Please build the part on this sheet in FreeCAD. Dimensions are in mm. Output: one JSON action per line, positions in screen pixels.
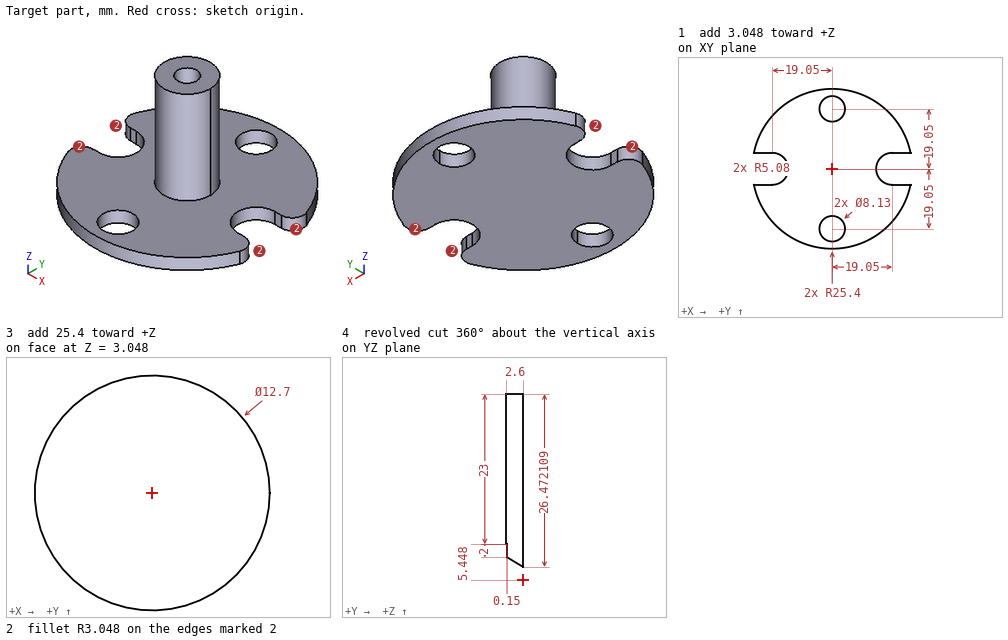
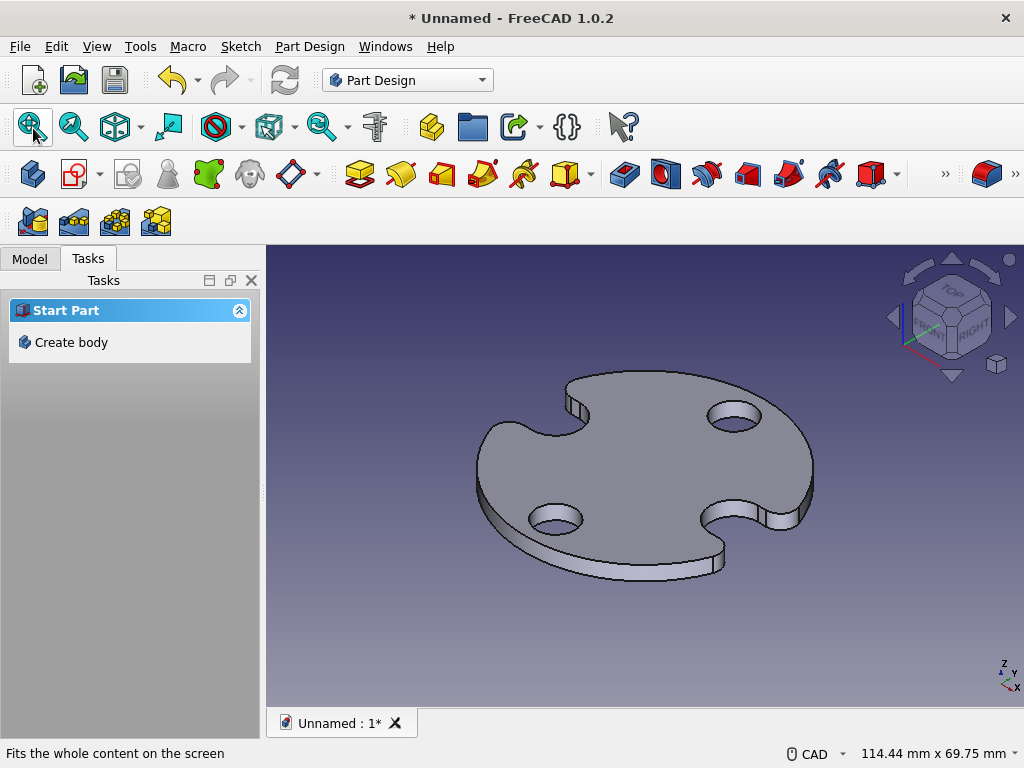
{"action": "left_click", "coordinate": [645, 467]}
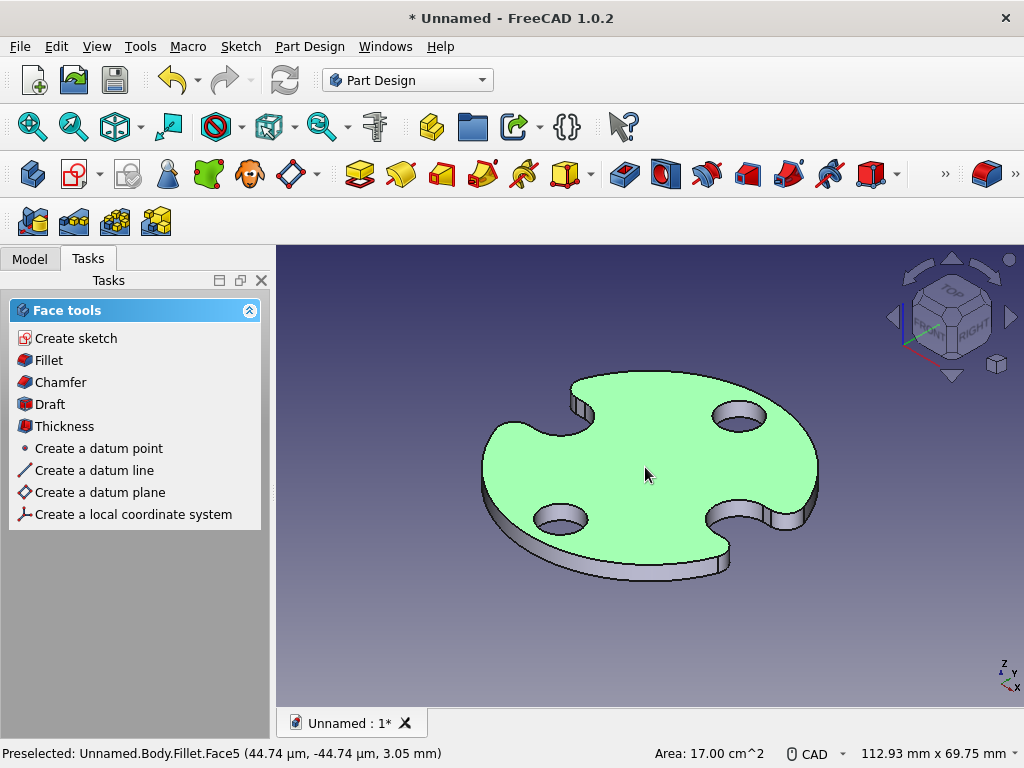
{"action": "left_click", "coordinate": [74, 174]}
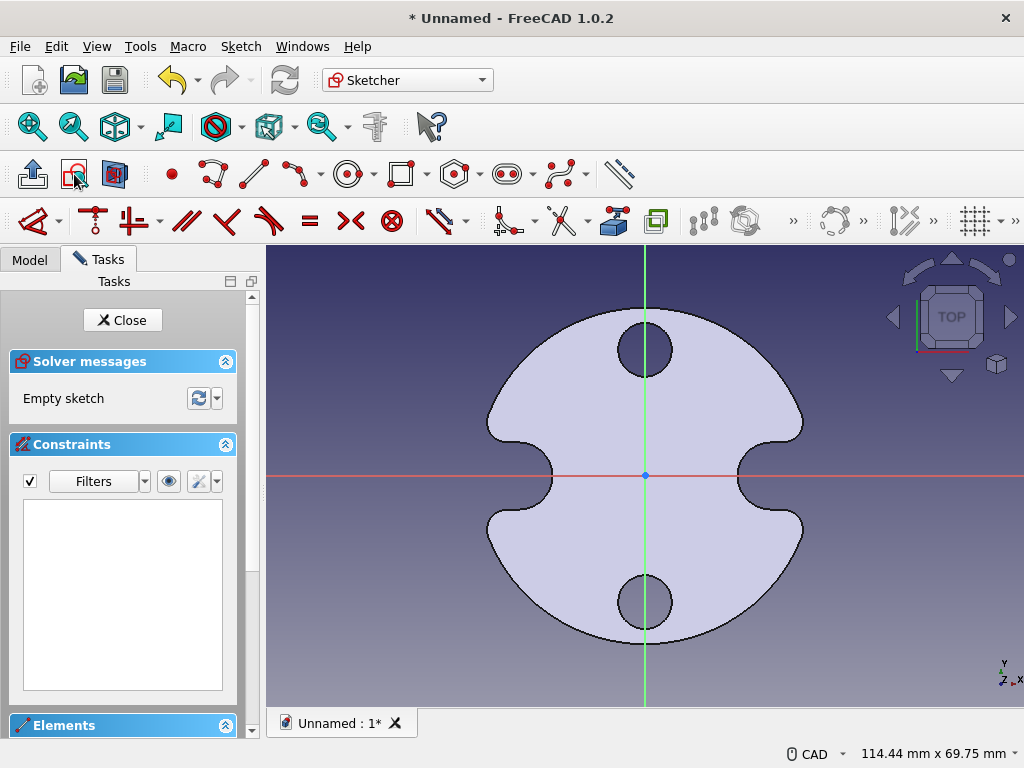
{"action": "scroll", "coordinate": [675, 476], "scroll_direction": "up", "scroll_amount": 6}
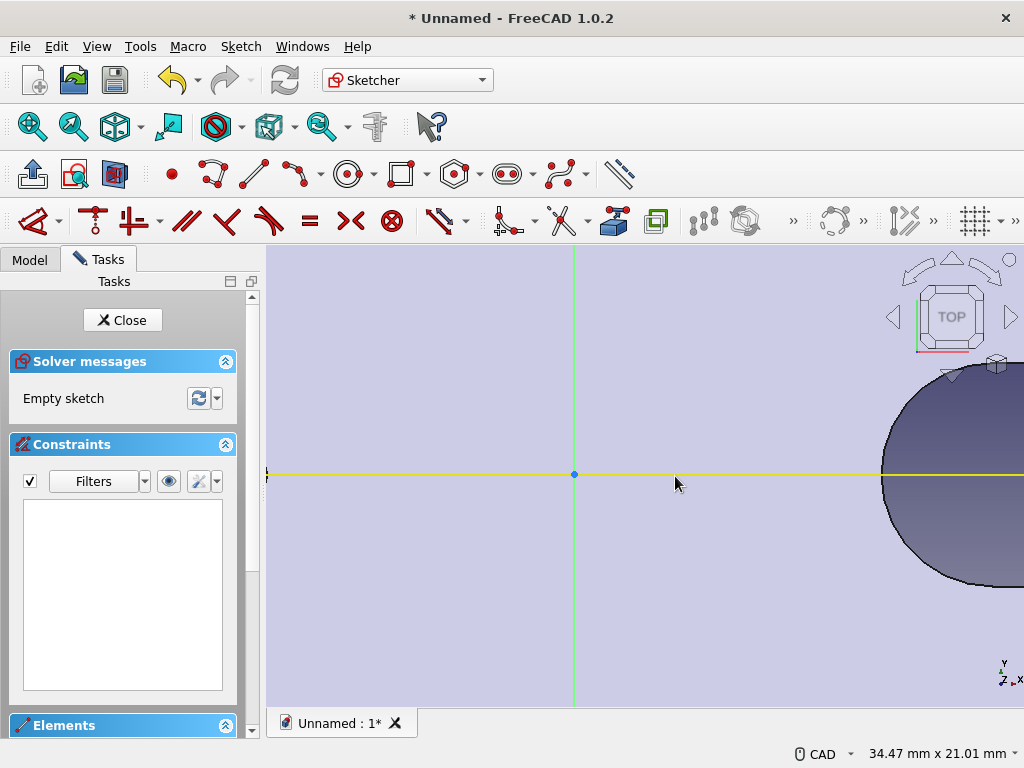
{"action": "left_click", "coordinate": [348, 174]}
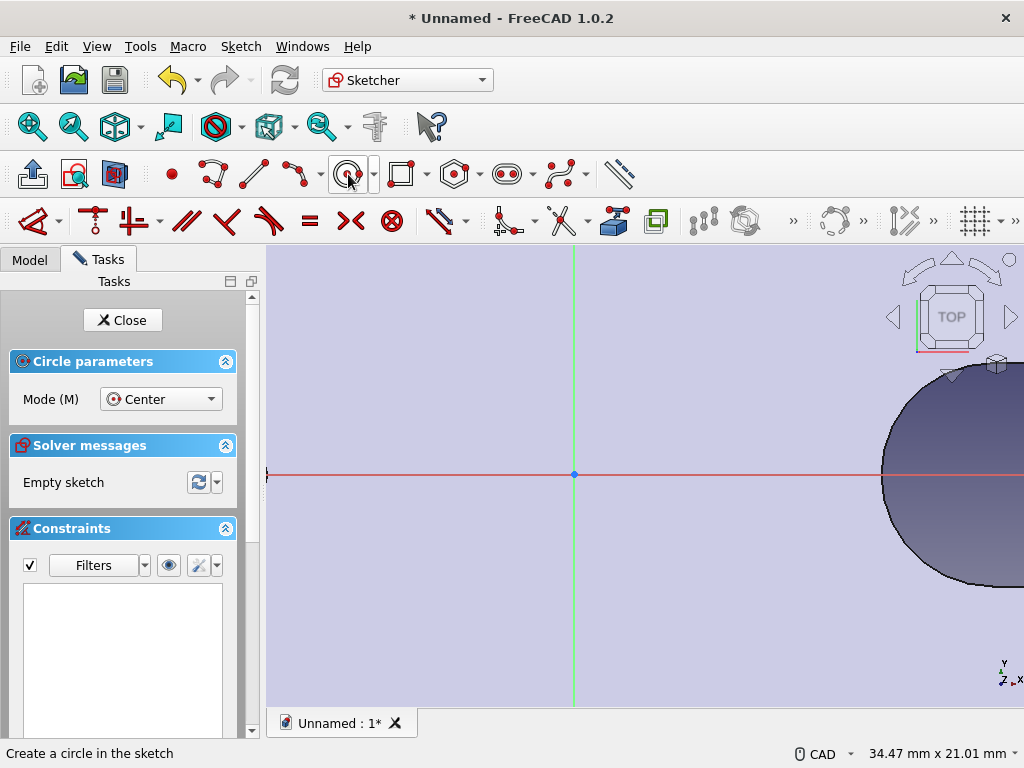
{"action": "left_click", "coordinate": [574, 475]}
{"action": "mouse_move", "coordinate": [673, 376]}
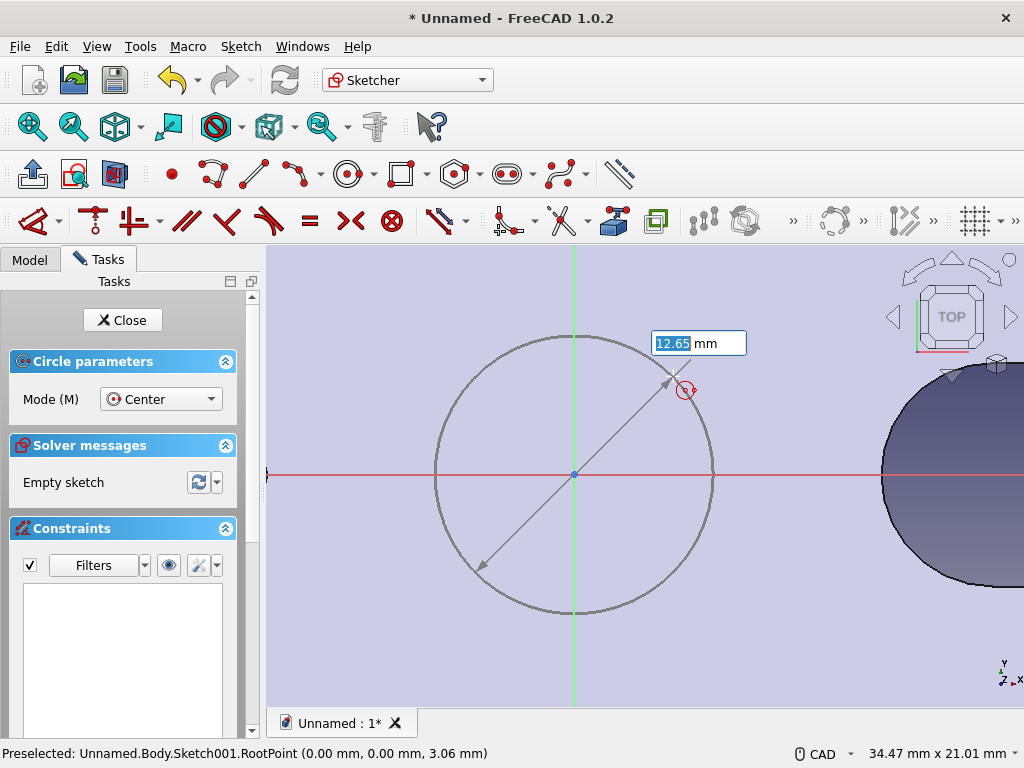
{"action": "type", "text": "12.7"}
{"action": "key", "text": "Return"}
{"action": "key", "text": "Escape"}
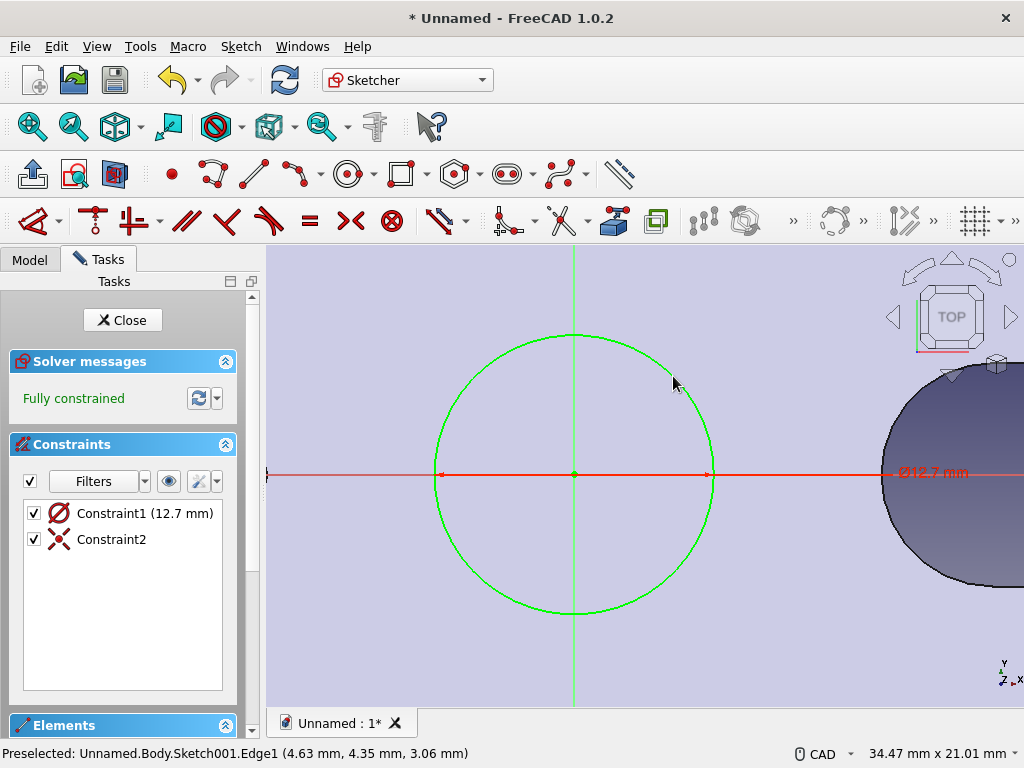
{"action": "left_click", "coordinate": [123, 320]}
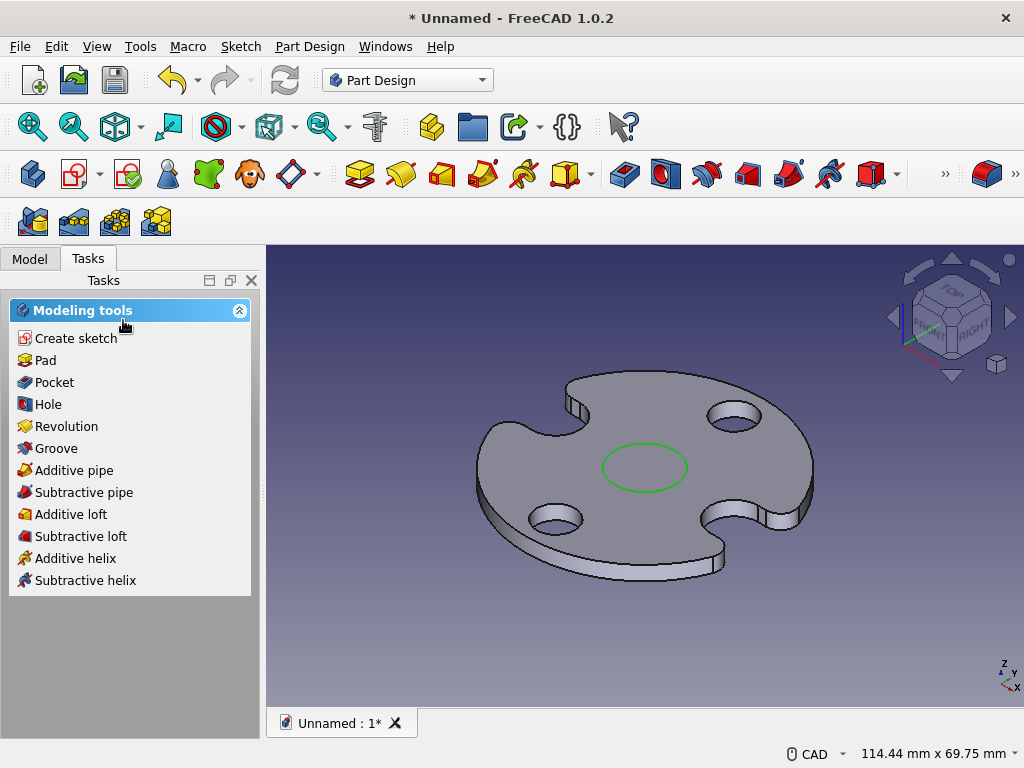
{"action": "left_click", "coordinate": [360, 174]}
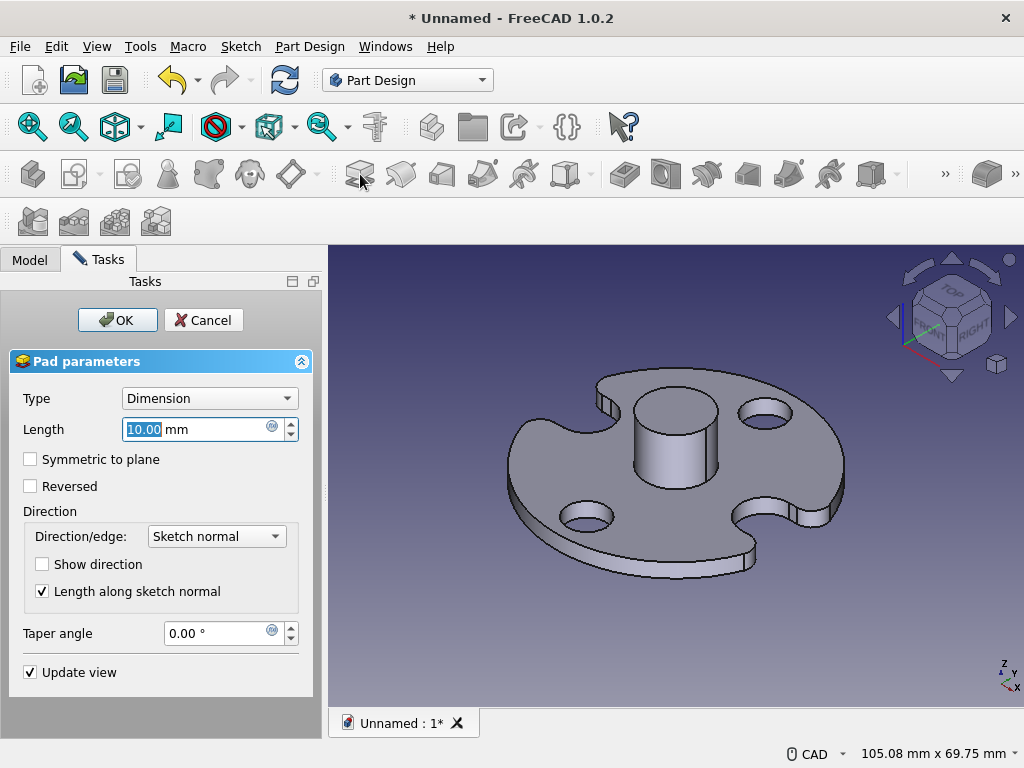
{"action": "type", "text": "25.4"}
{"action": "key", "text": "Tab"}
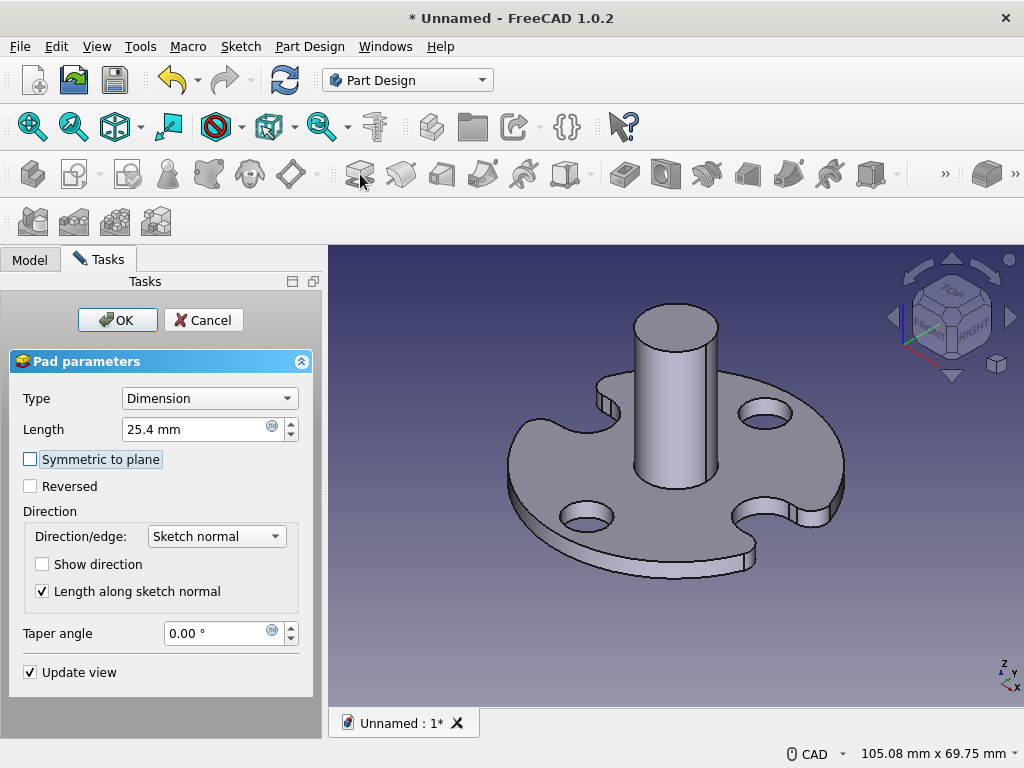
{"action": "left_click", "coordinate": [118, 320]}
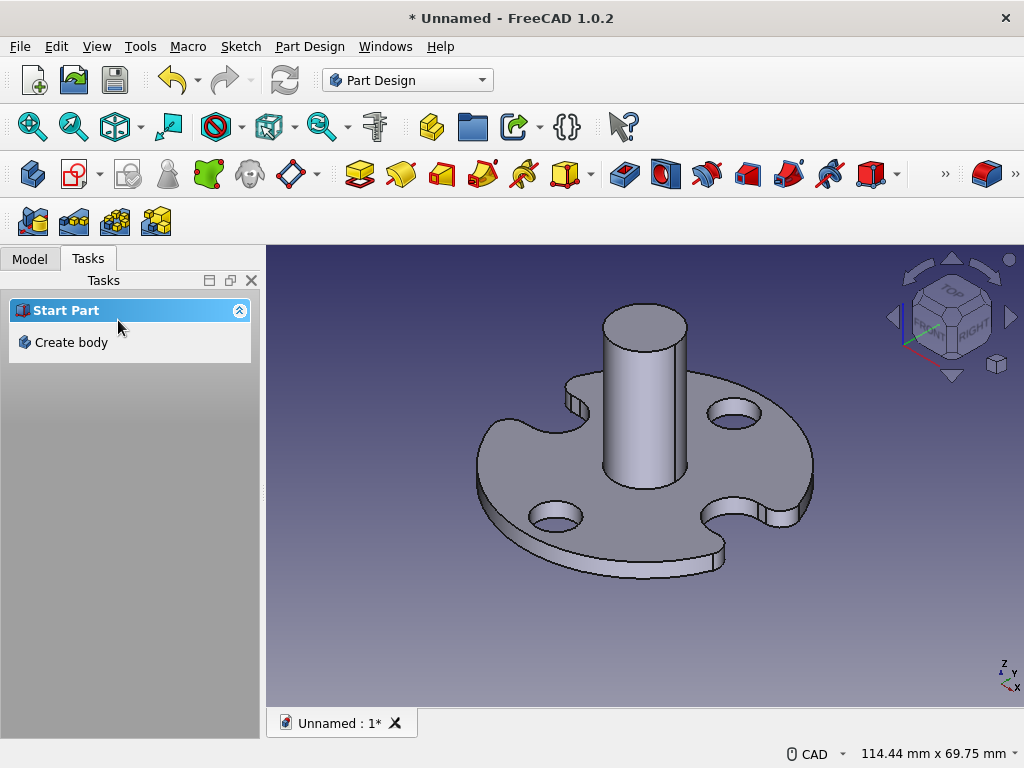
{"action": "left_click", "coordinate": [33, 128]}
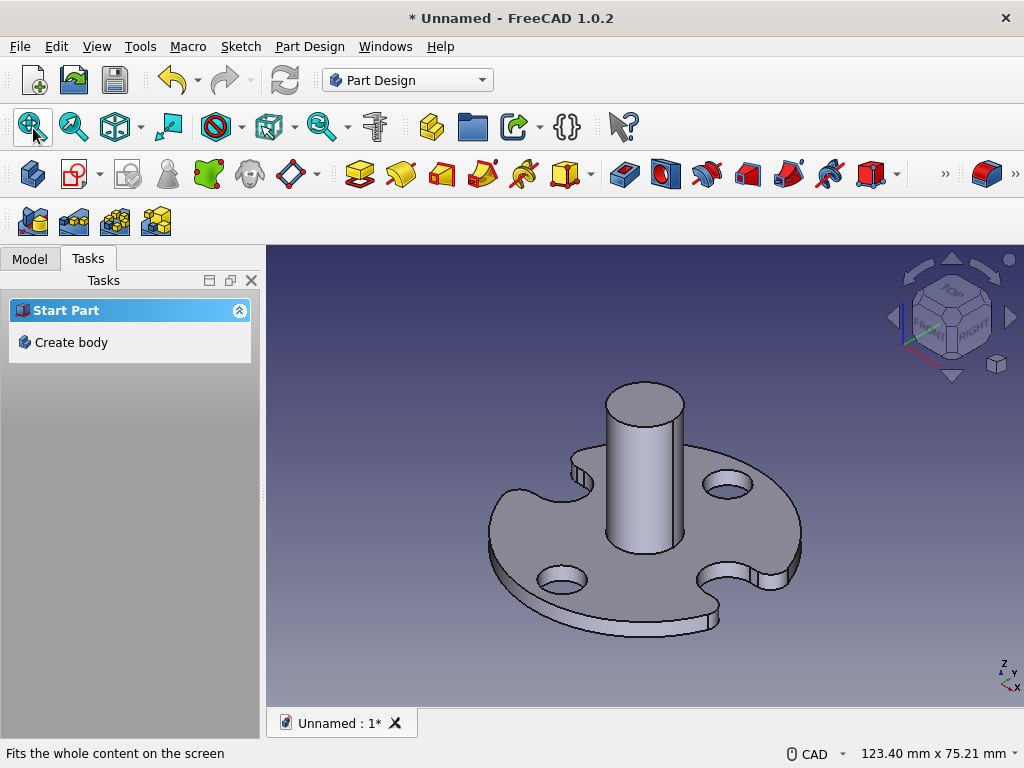
{"action": "left_click", "coordinate": [74, 174]}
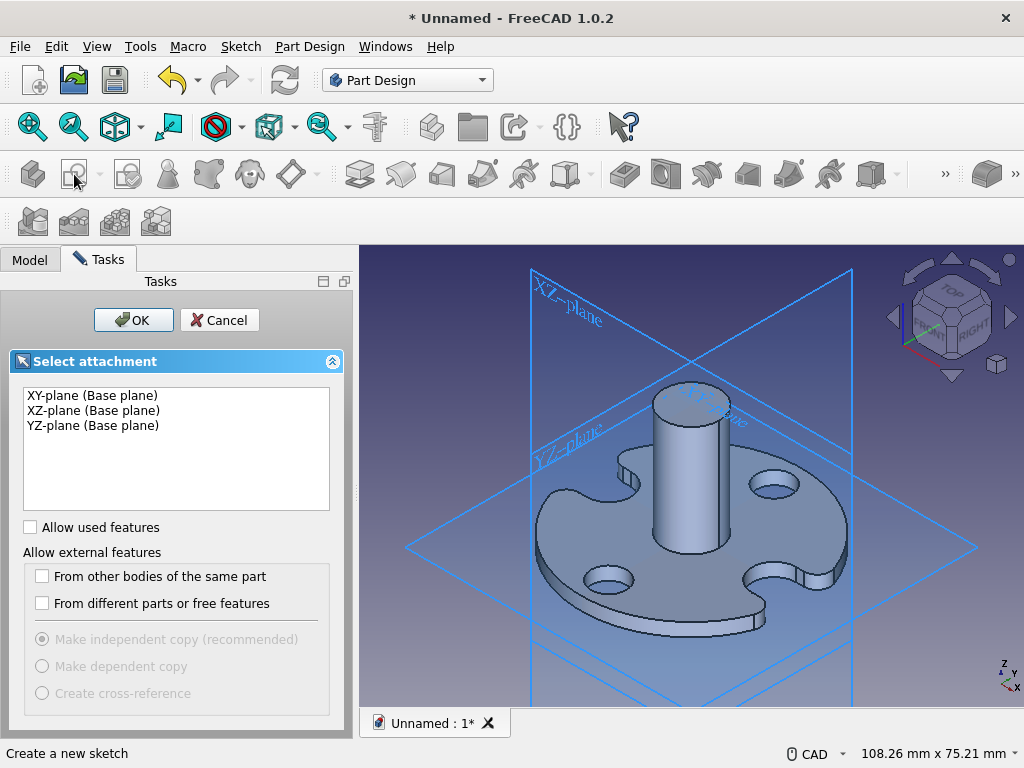
{"action": "left_click", "coordinate": [84, 426]}